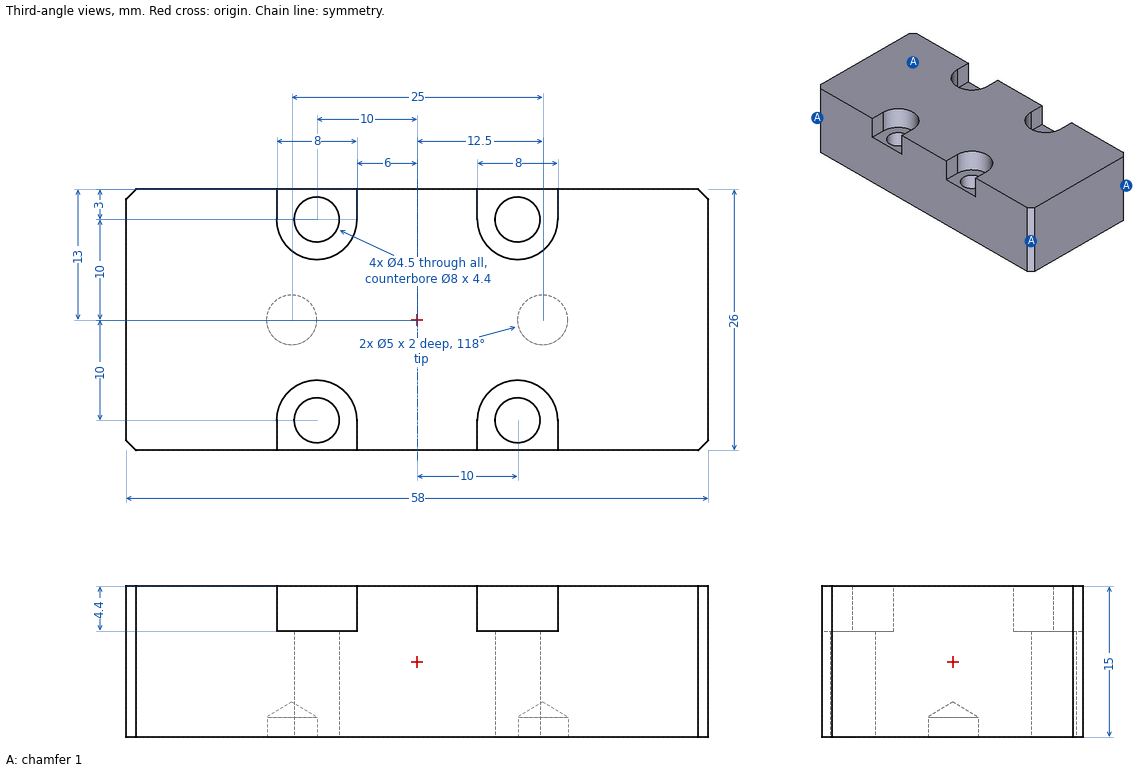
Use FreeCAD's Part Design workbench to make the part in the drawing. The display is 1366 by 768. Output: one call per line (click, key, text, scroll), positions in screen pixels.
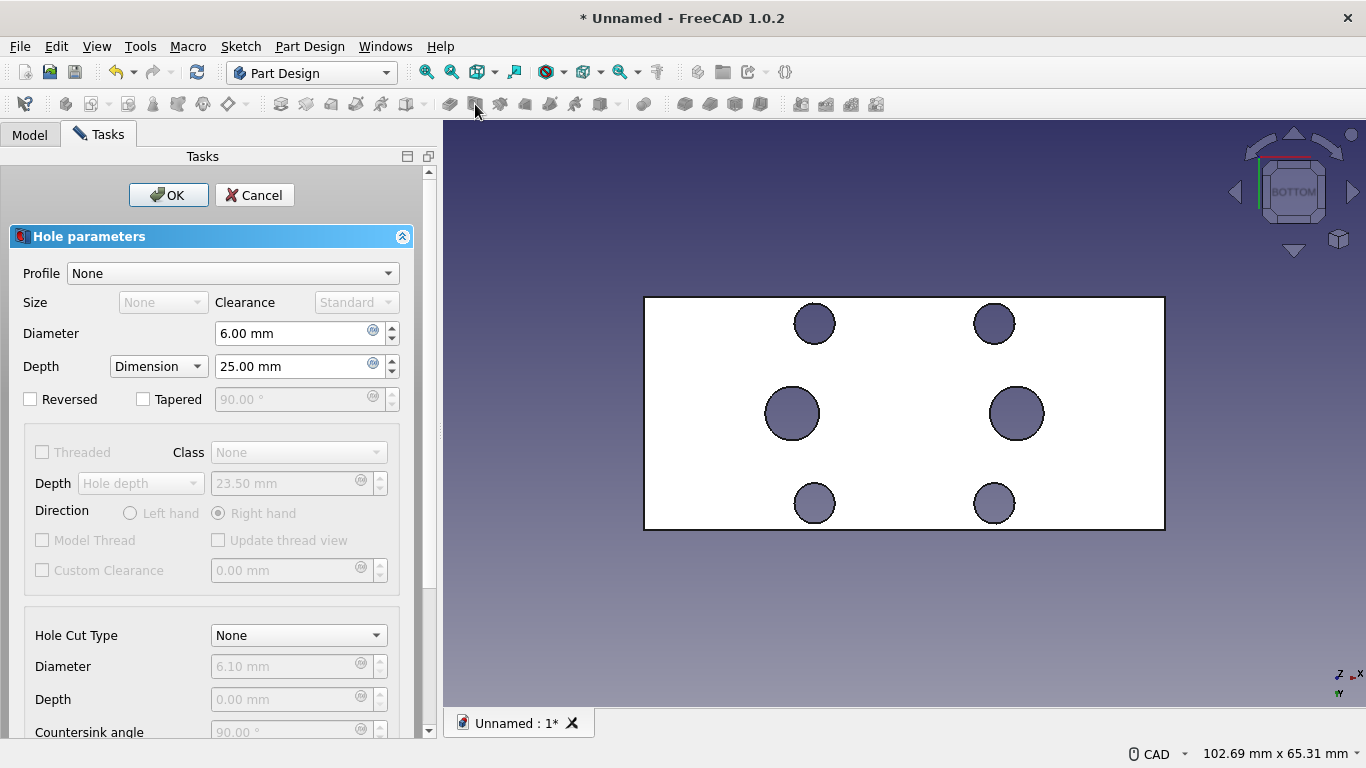
triple_click(300, 334)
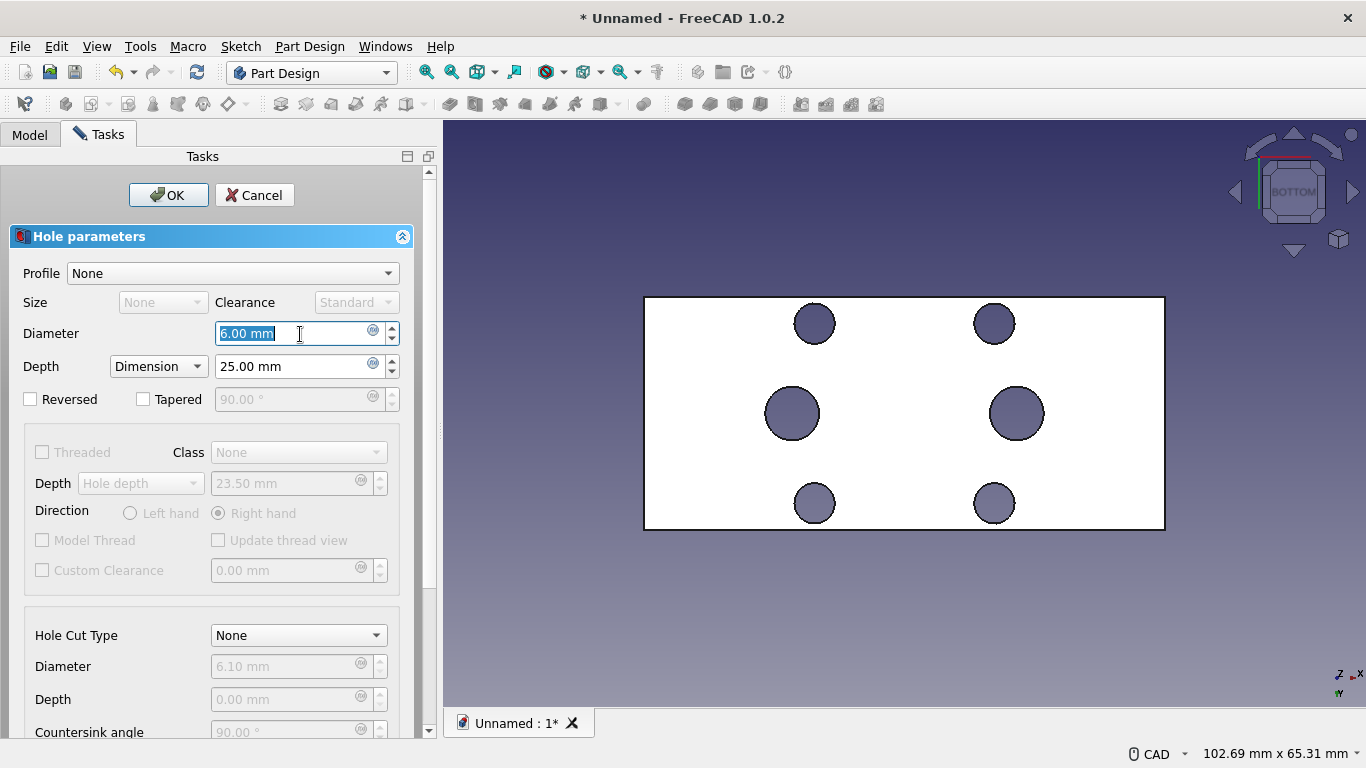
text(5)
key(Tab)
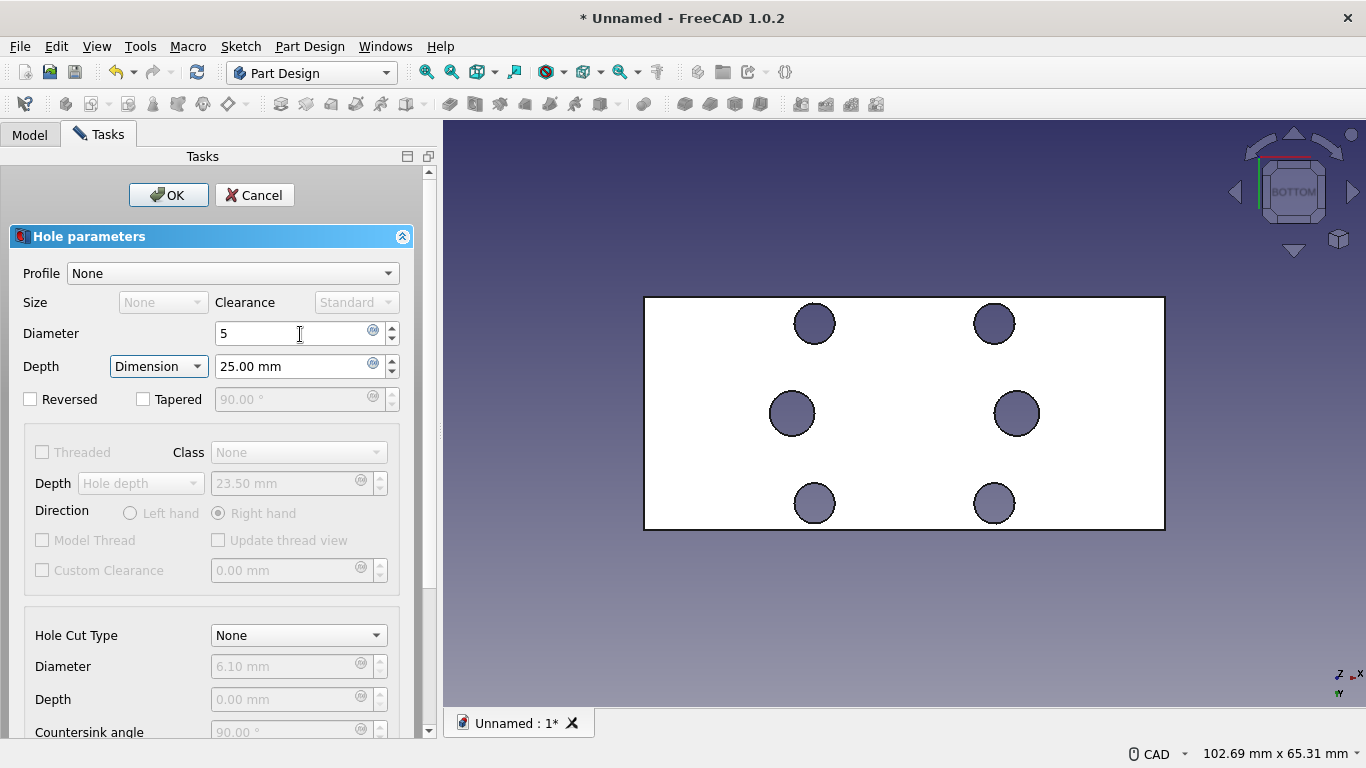
triple_click(300, 366)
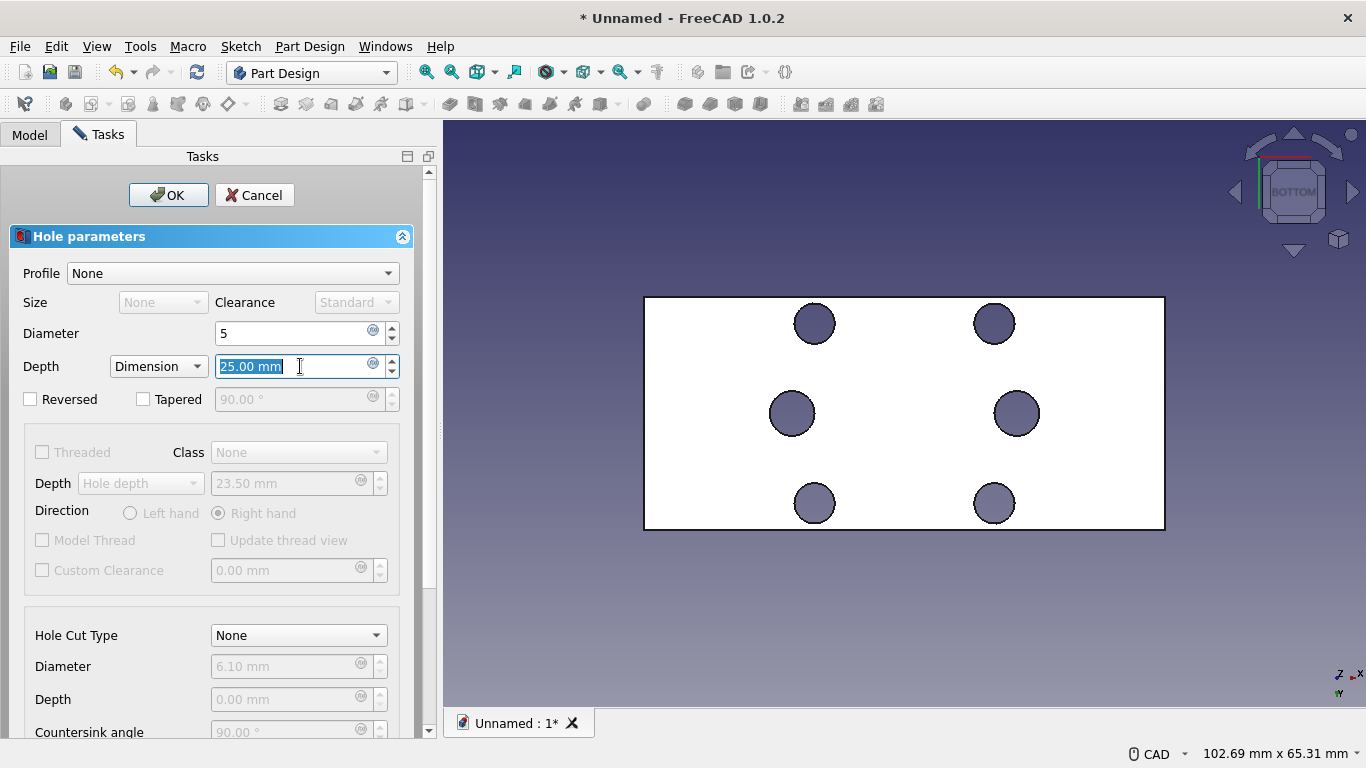
text(2)
key(Tab)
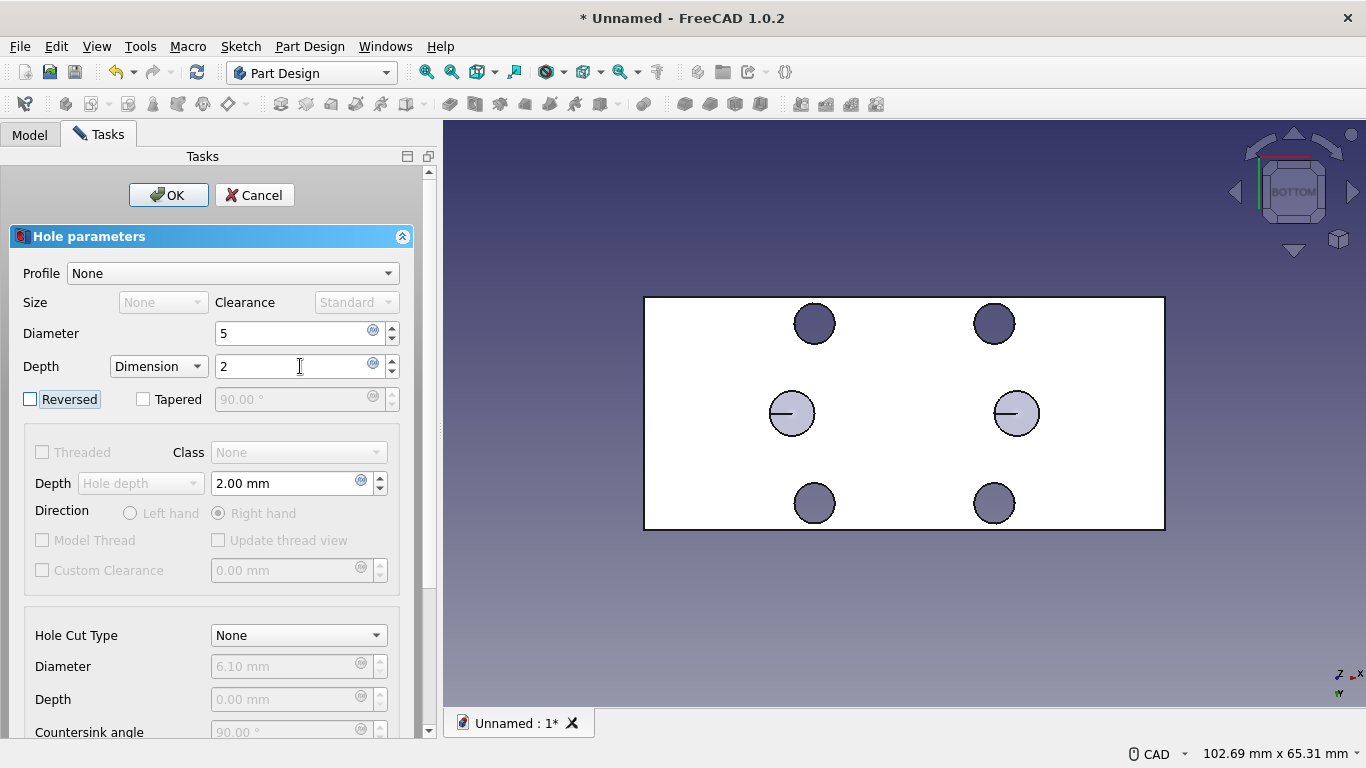
click(169, 195)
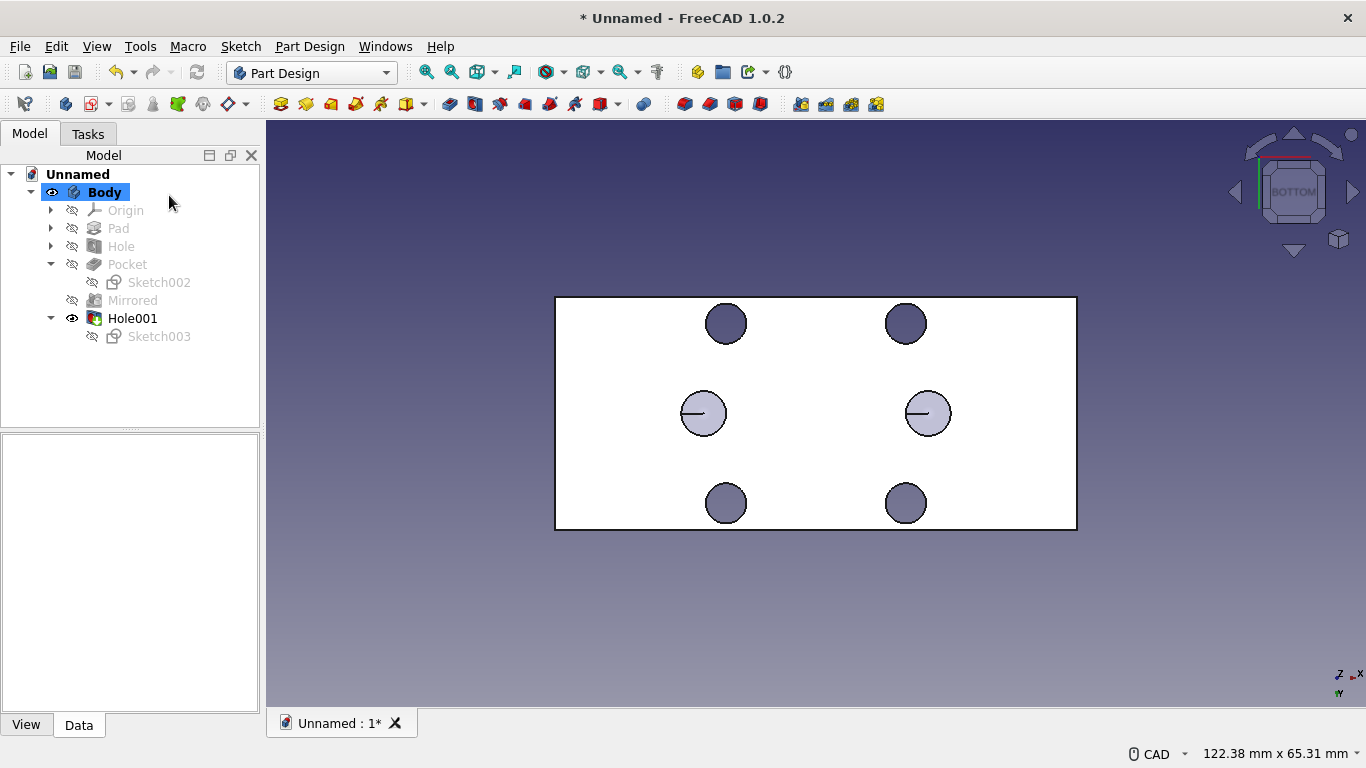
key(0)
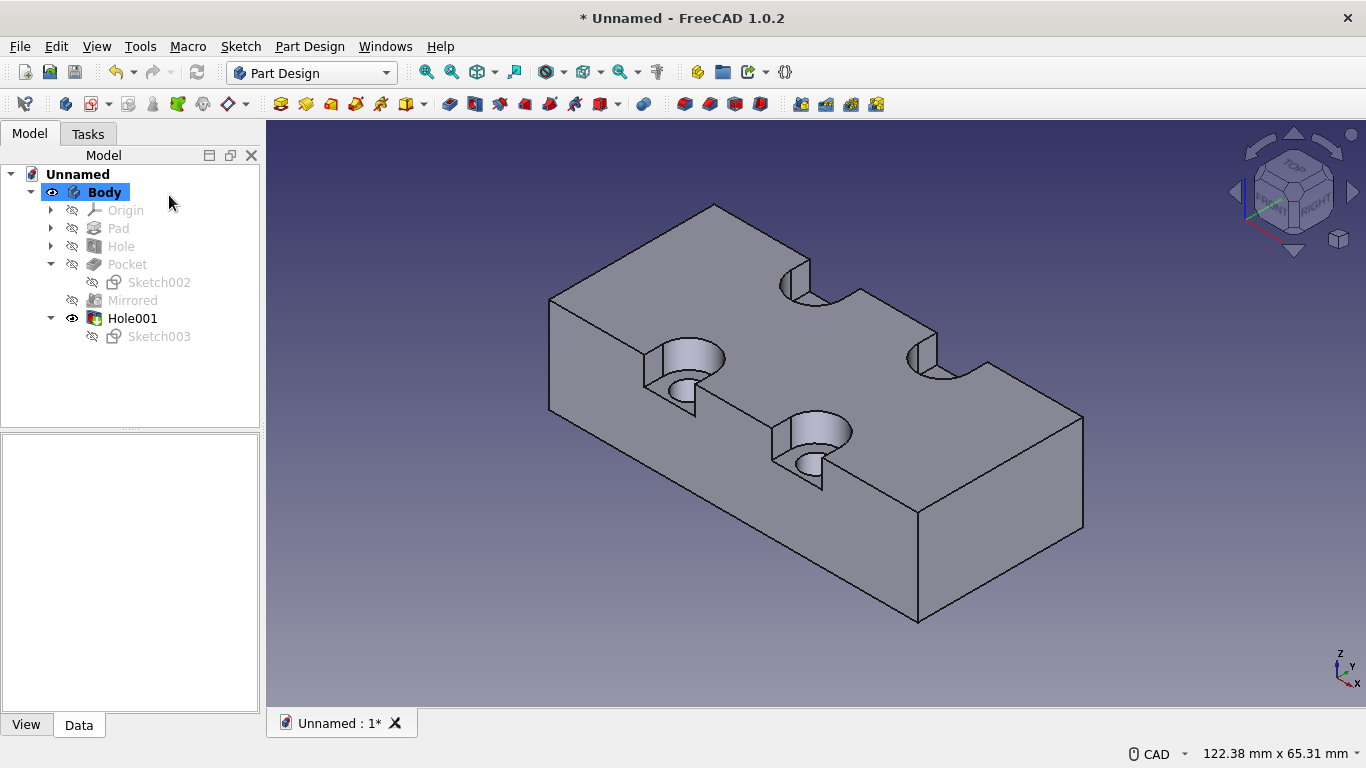
click(918, 567)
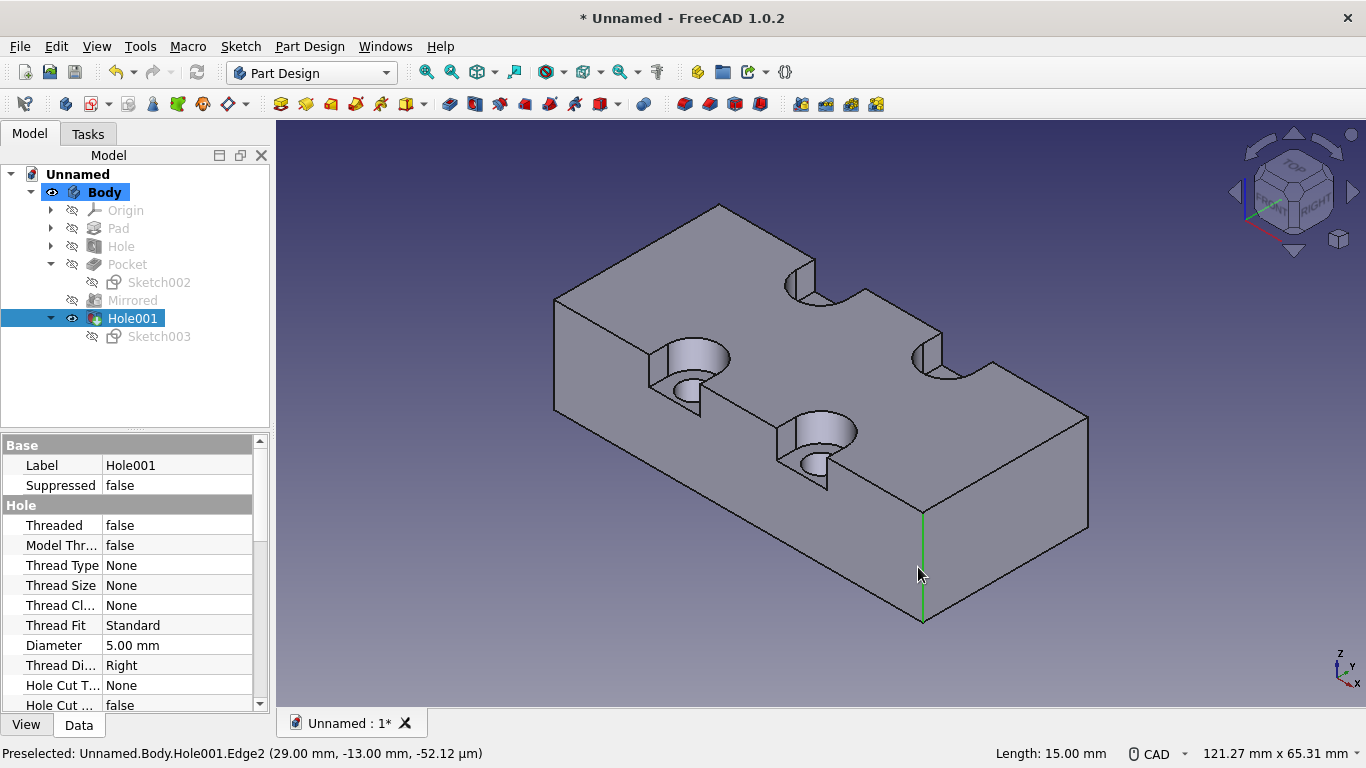
key(2)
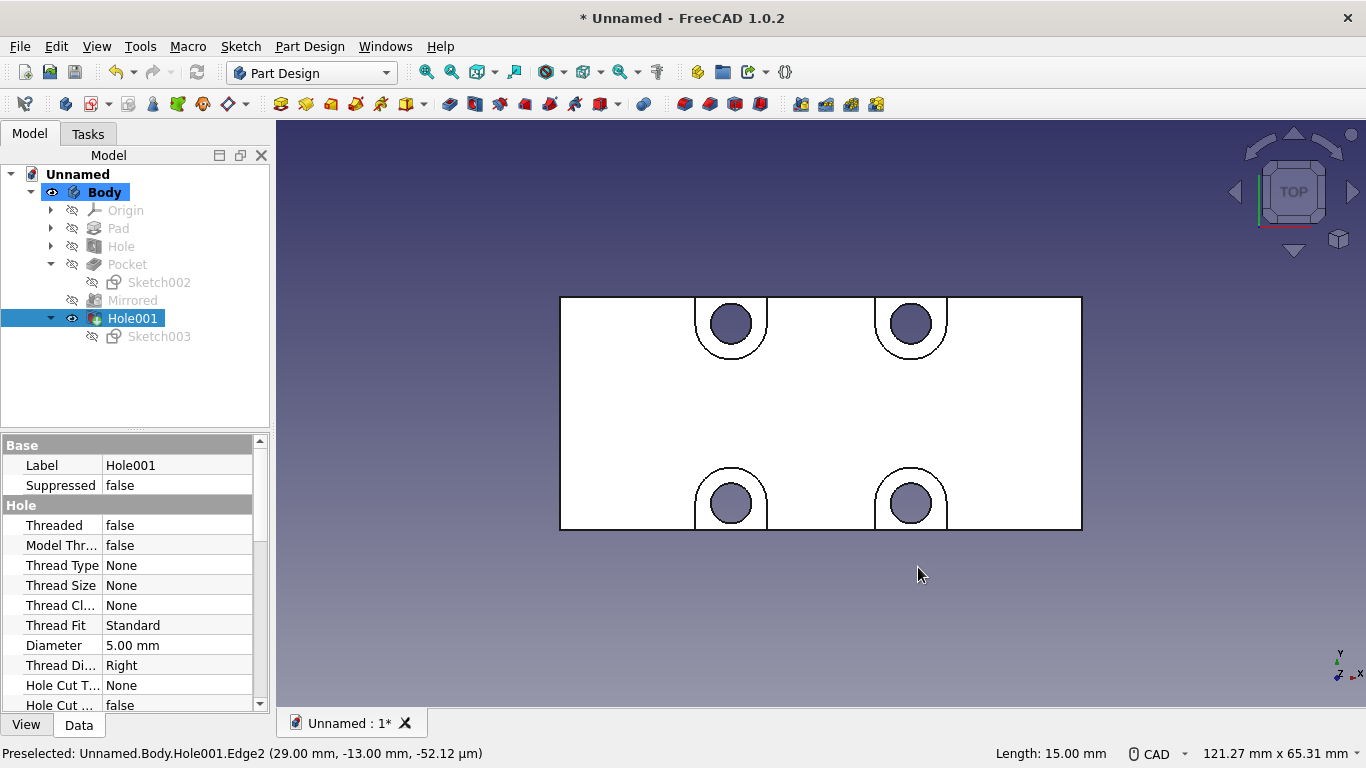
key(1)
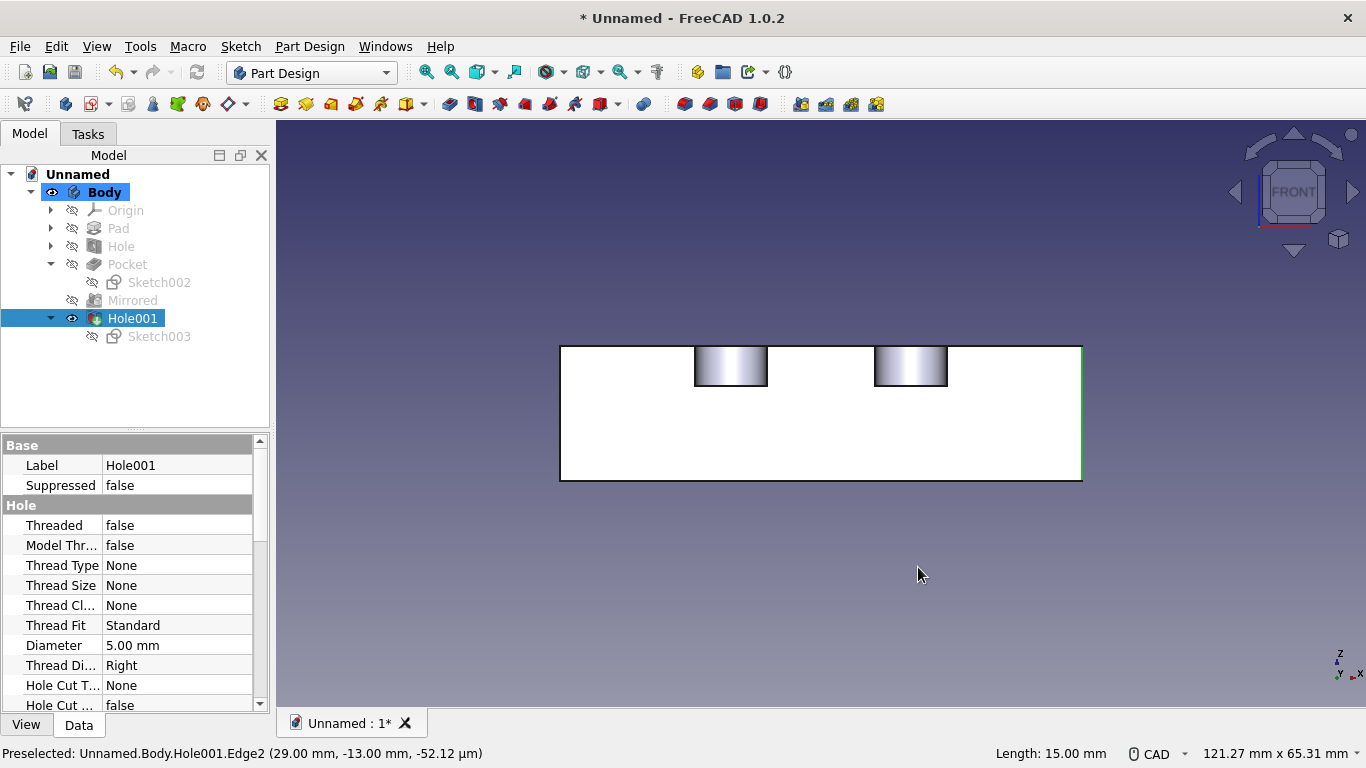
click(560, 412, ctrl)